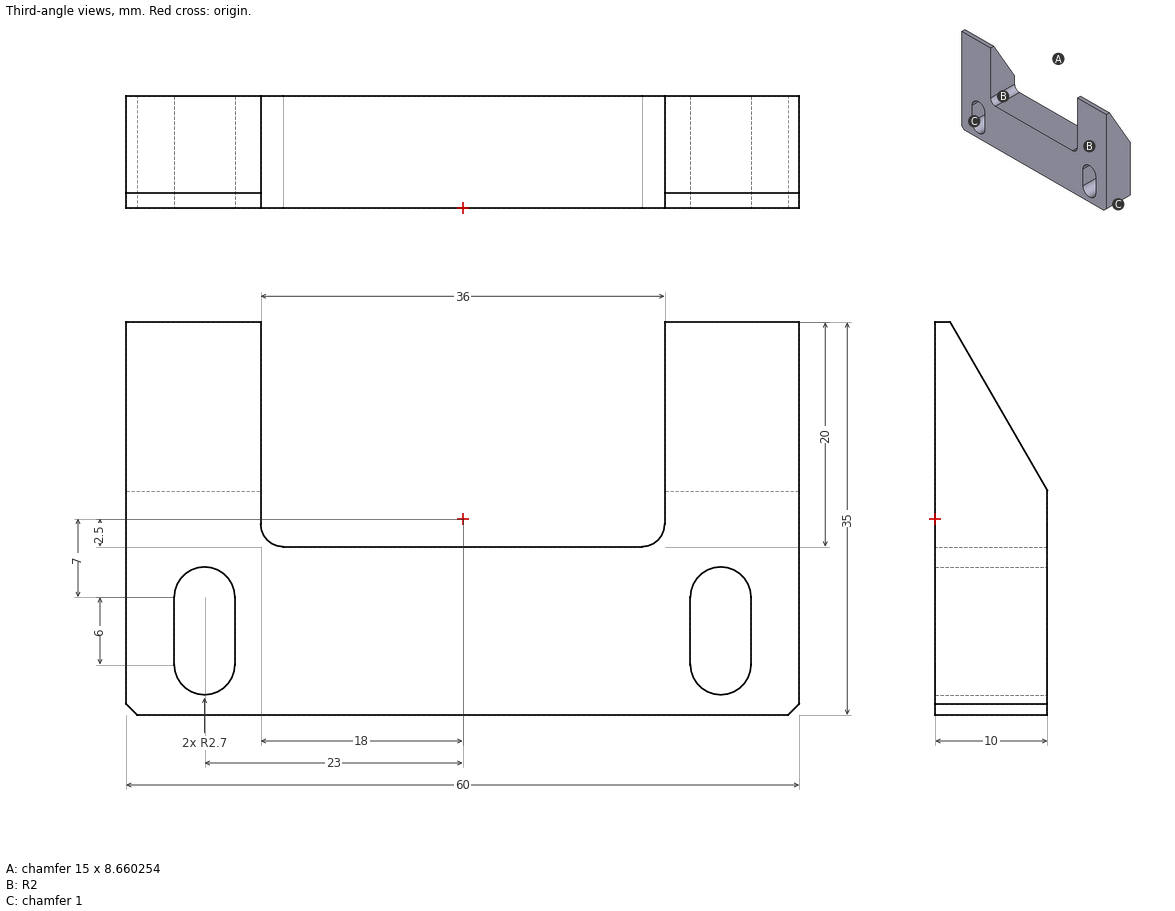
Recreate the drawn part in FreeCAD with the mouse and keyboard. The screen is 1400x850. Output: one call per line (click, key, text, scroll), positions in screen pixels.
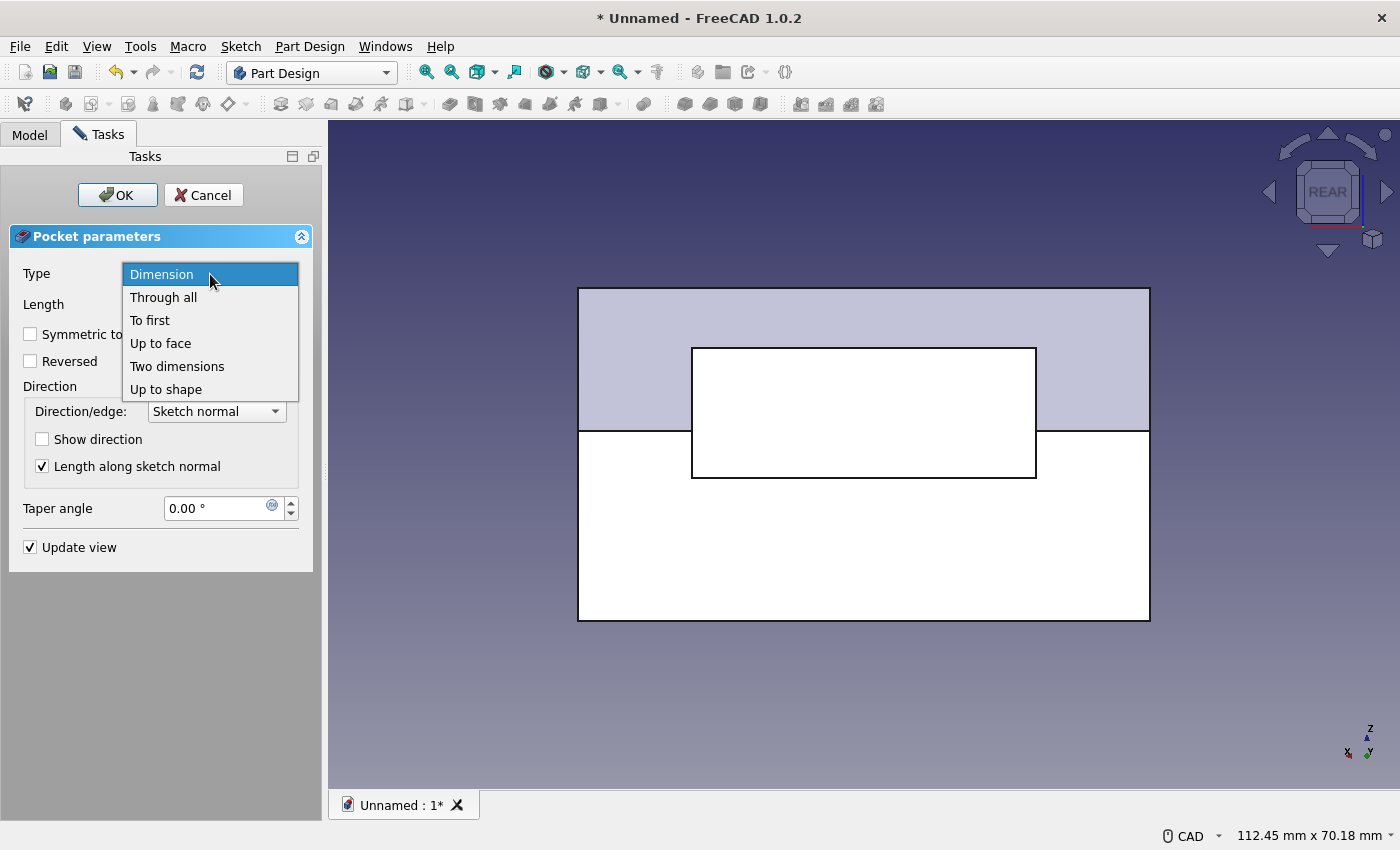
click(208, 298)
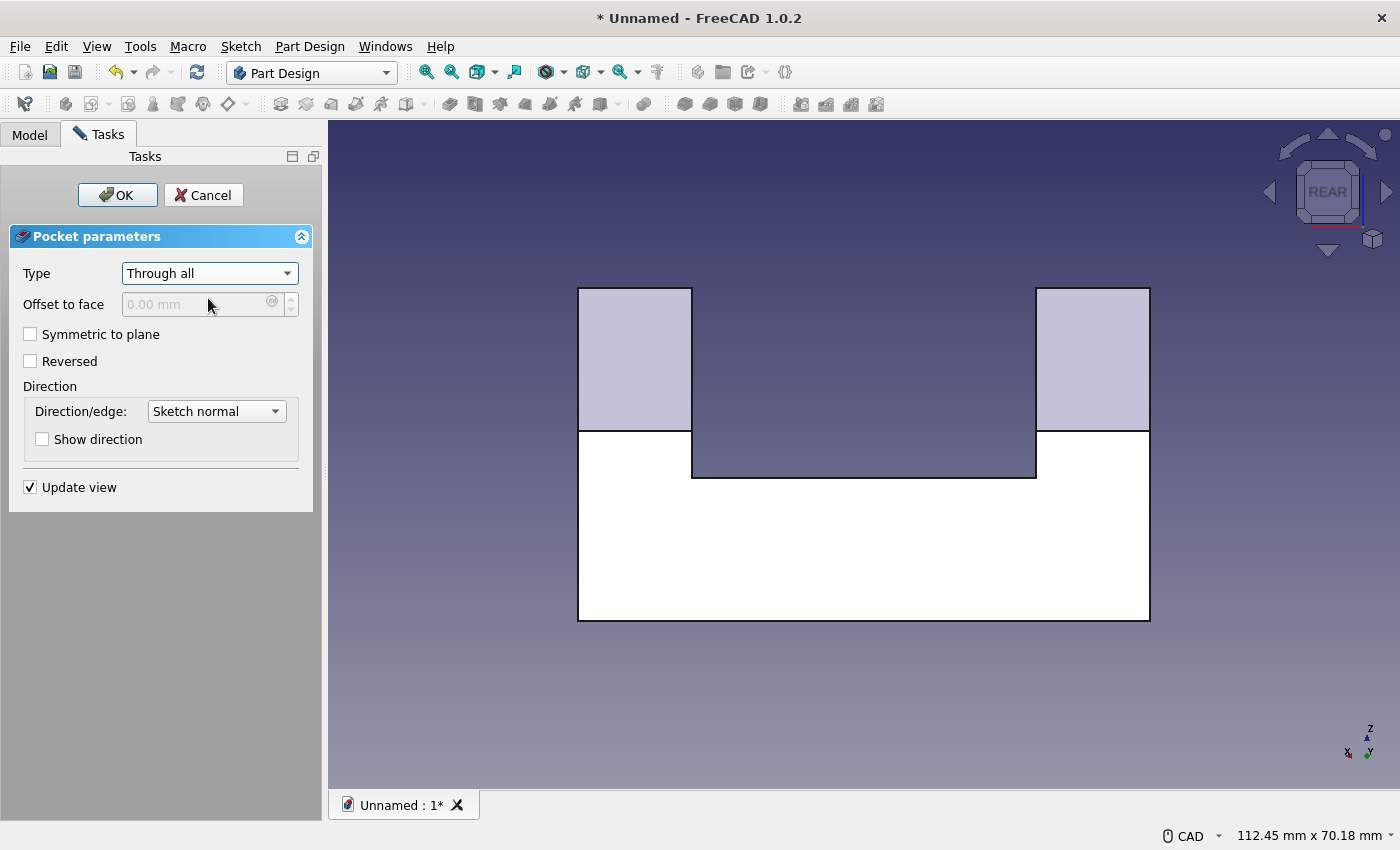
click(118, 195)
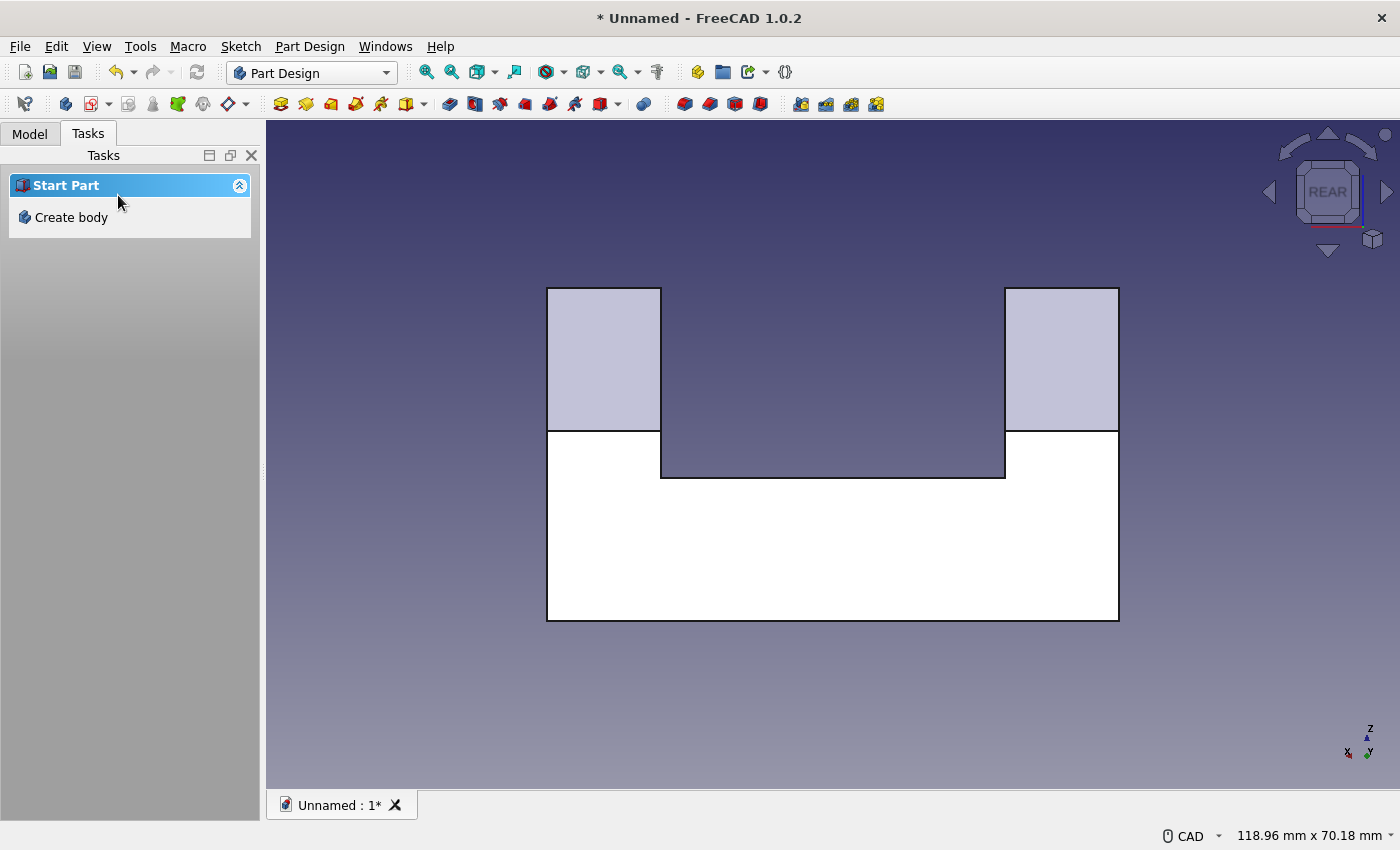
key(0)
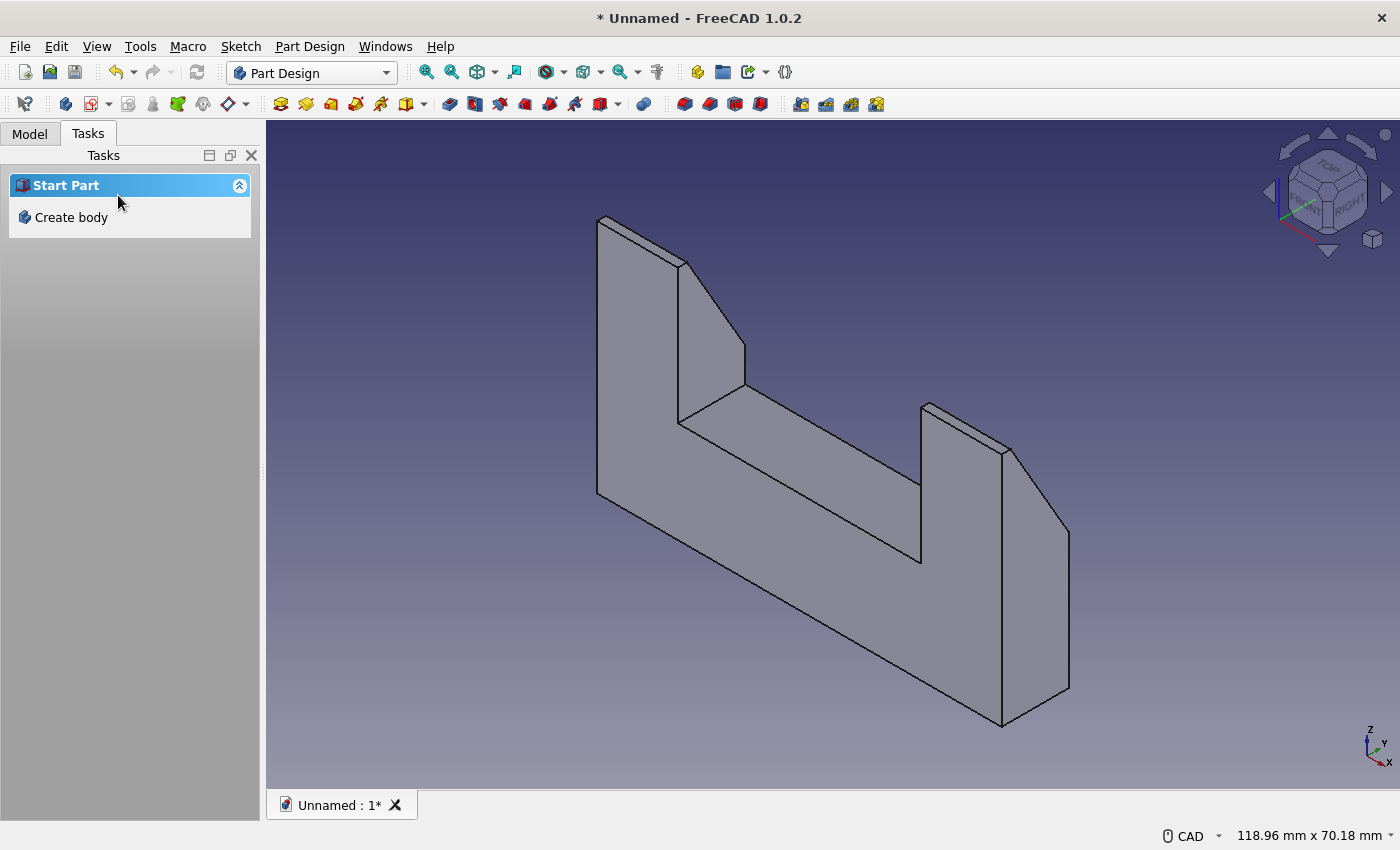
key(2)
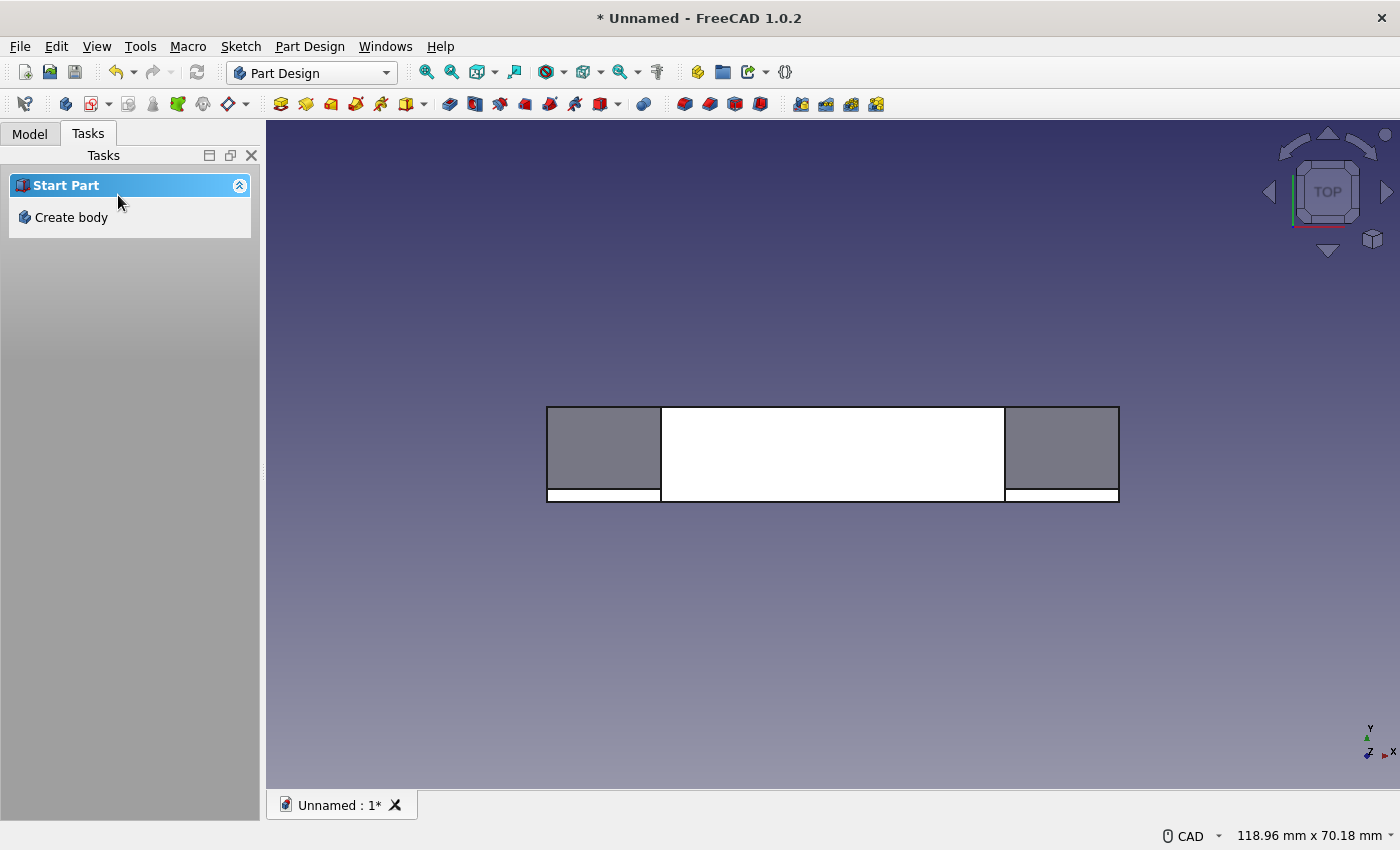
key(1)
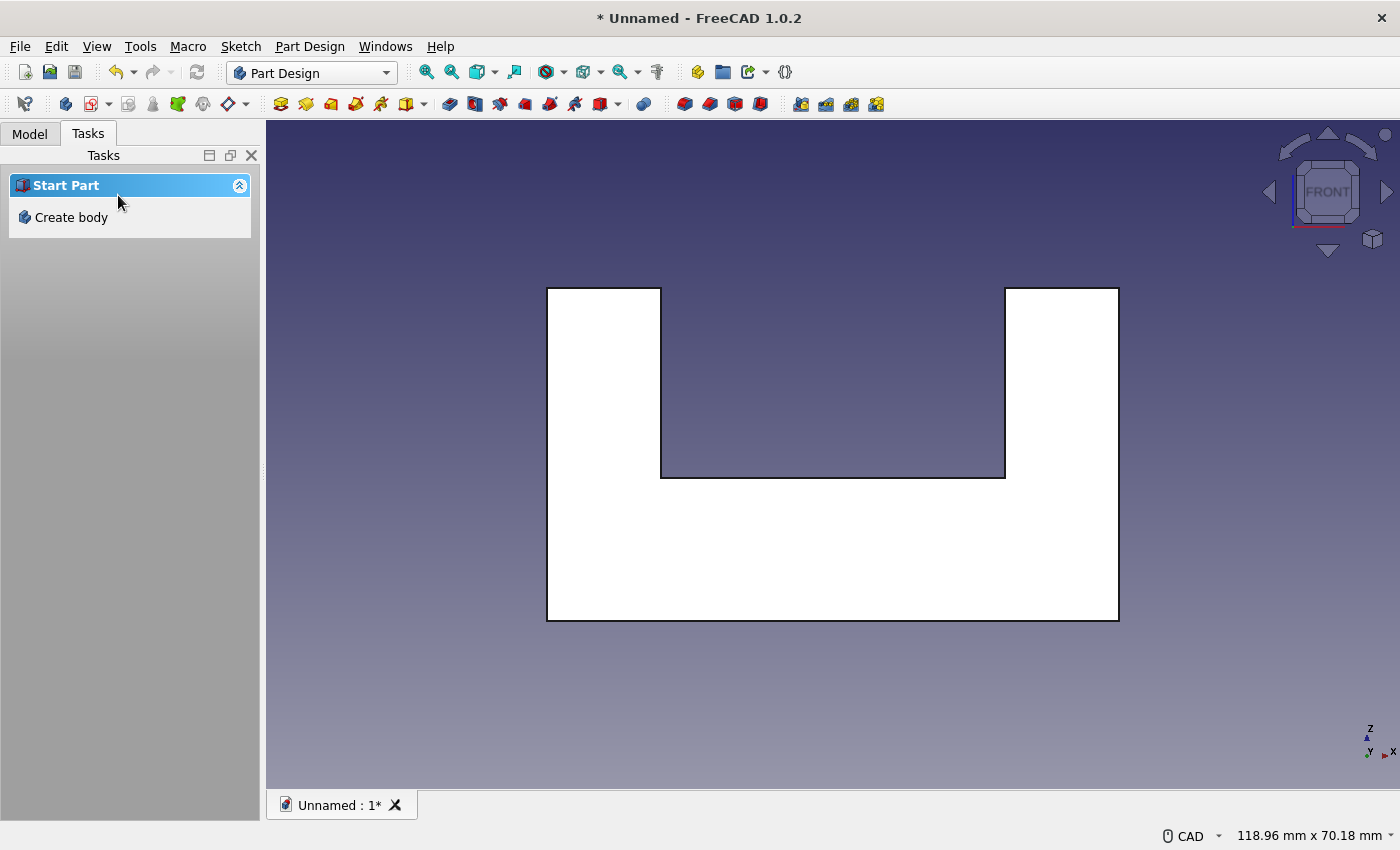
key(3)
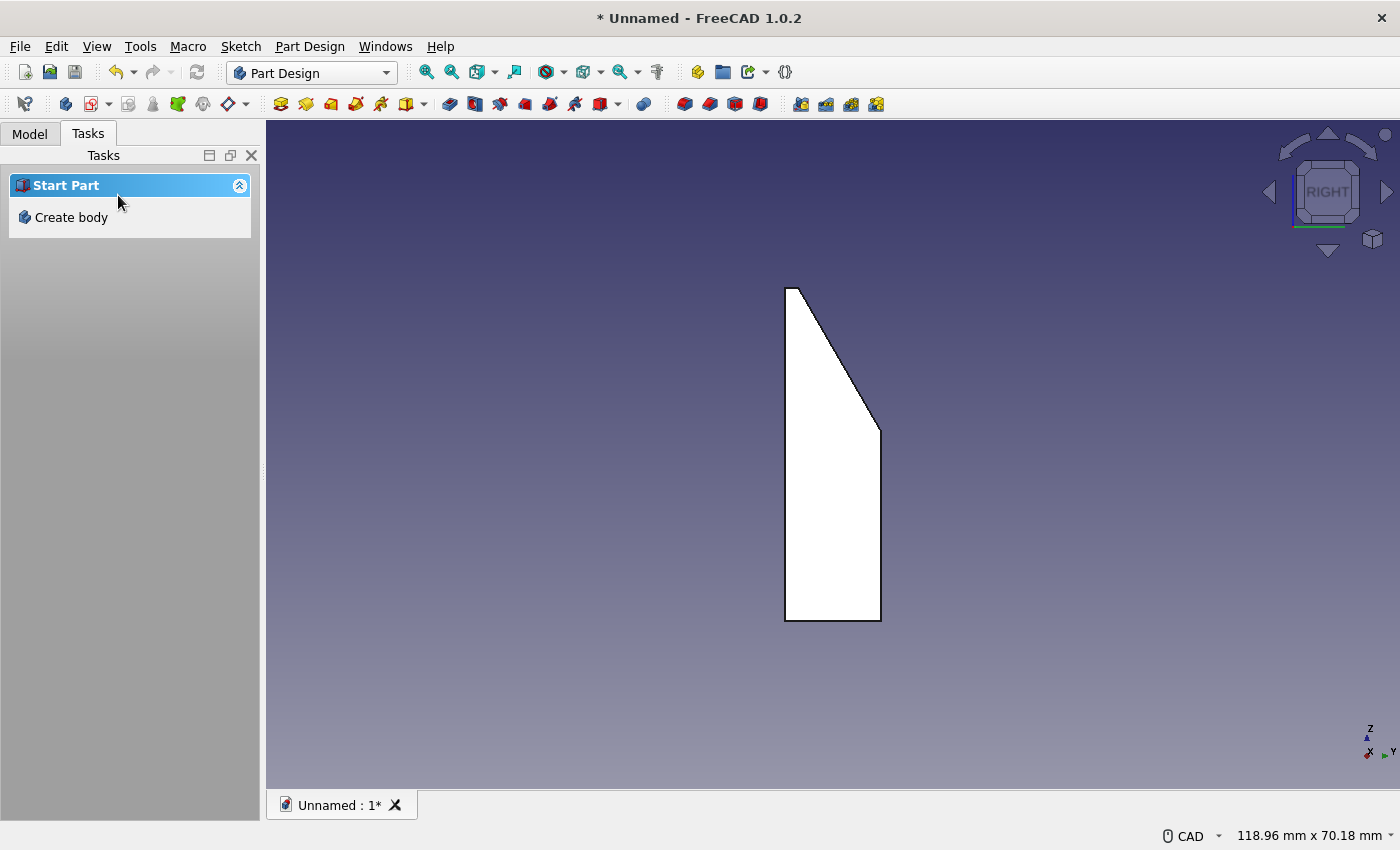
key(5)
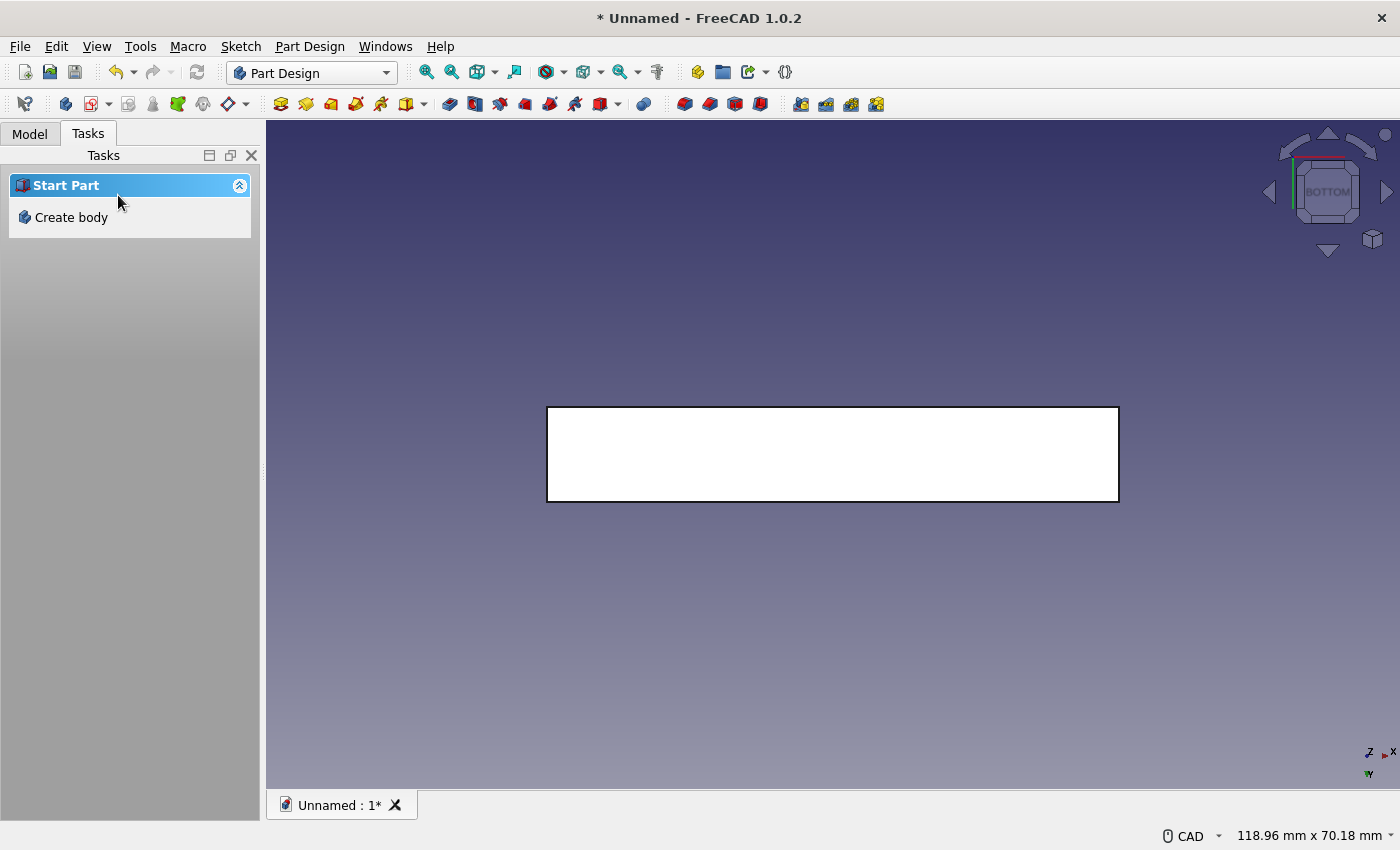
key(4)